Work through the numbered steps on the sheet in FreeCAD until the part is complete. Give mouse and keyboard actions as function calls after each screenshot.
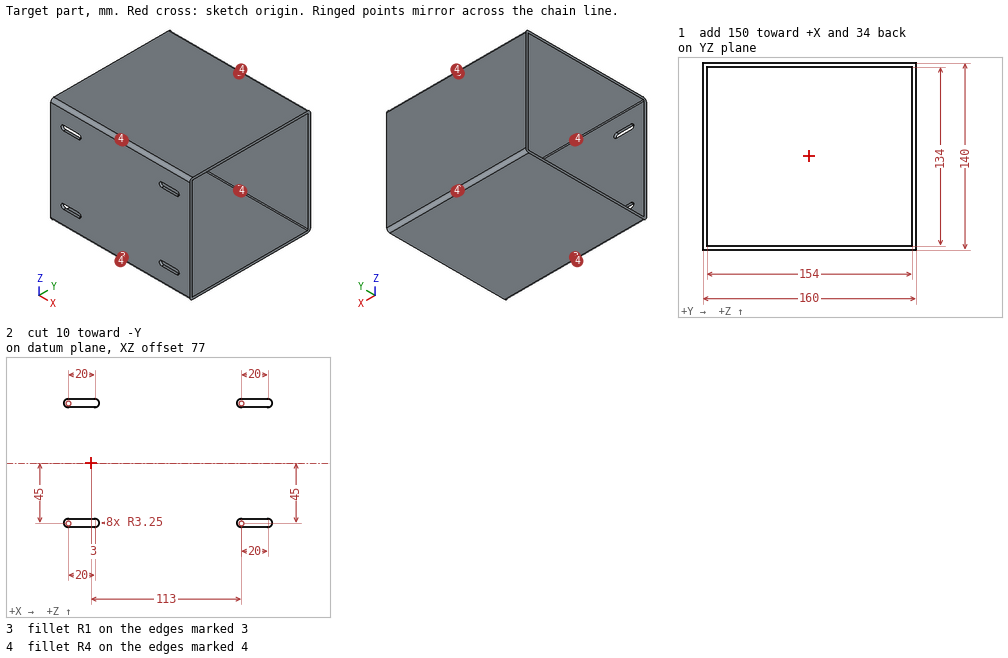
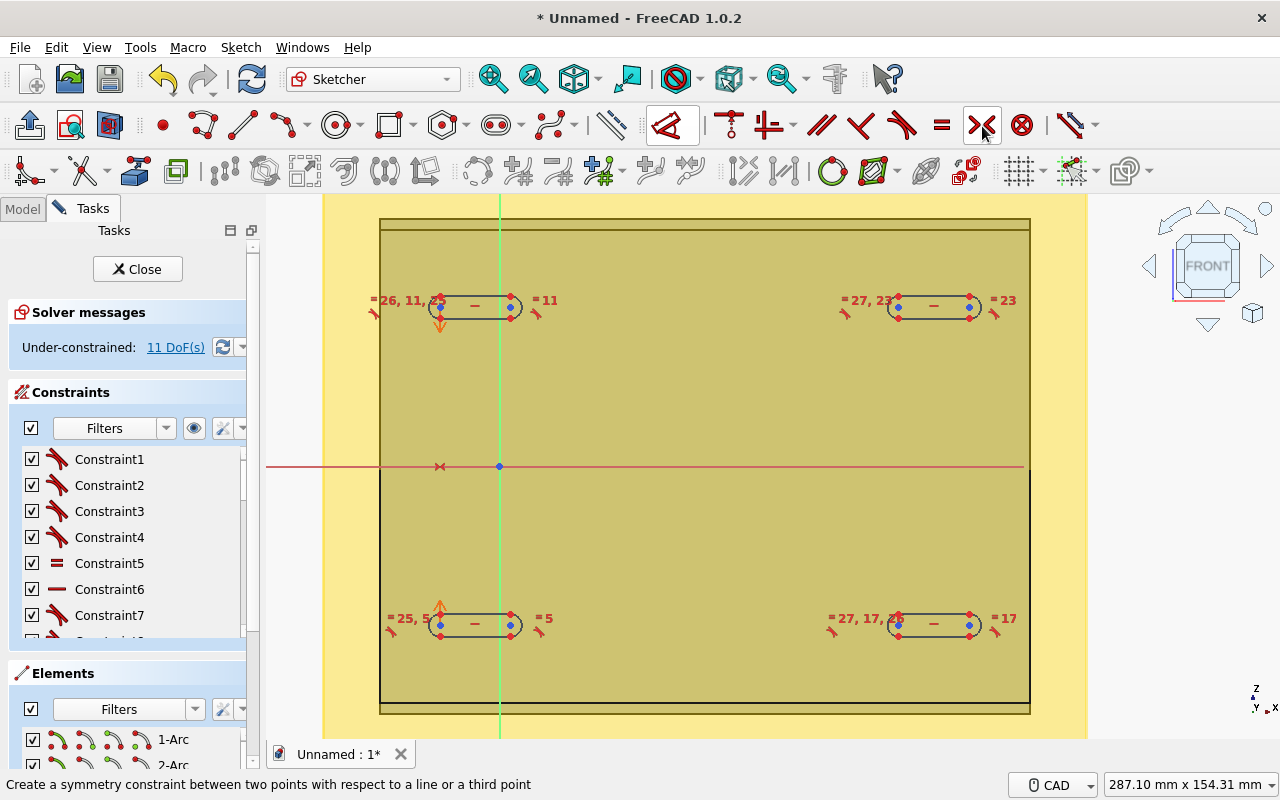
click(899, 625)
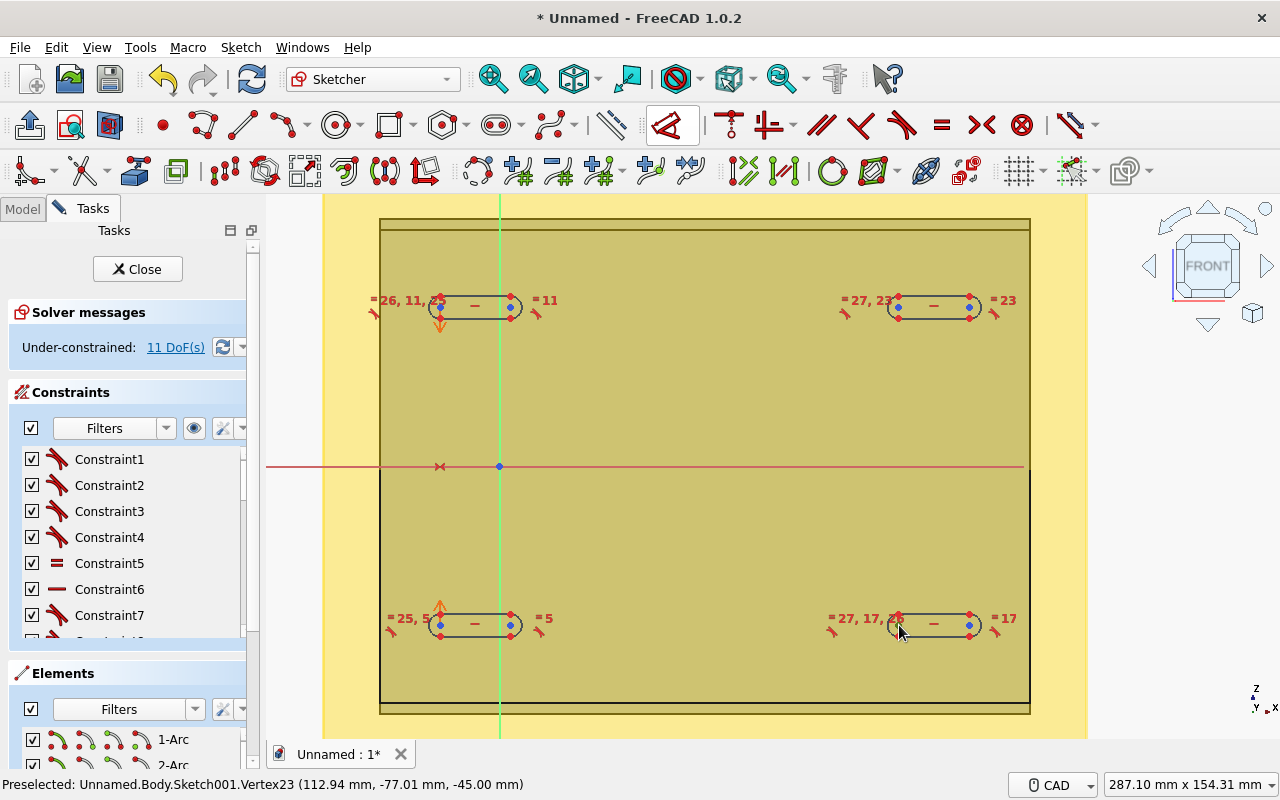
click(899, 308)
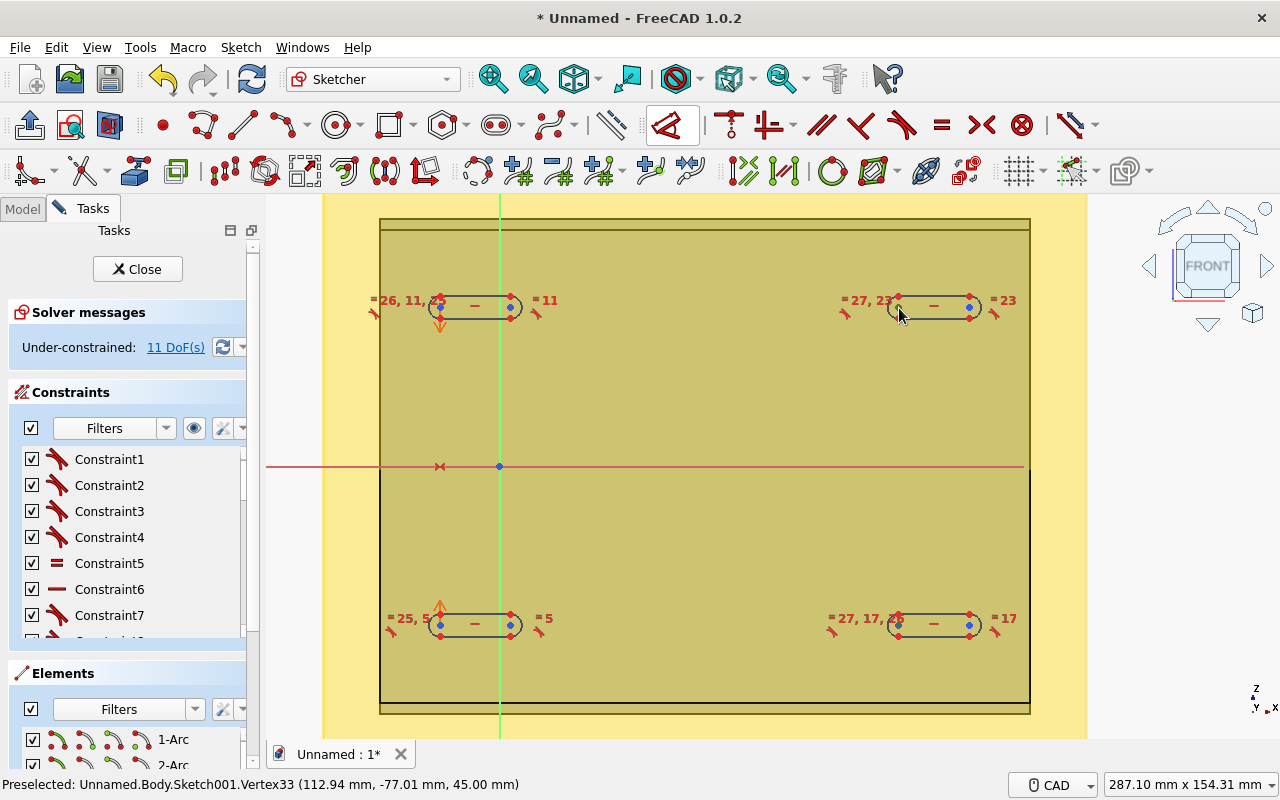
click(353, 466)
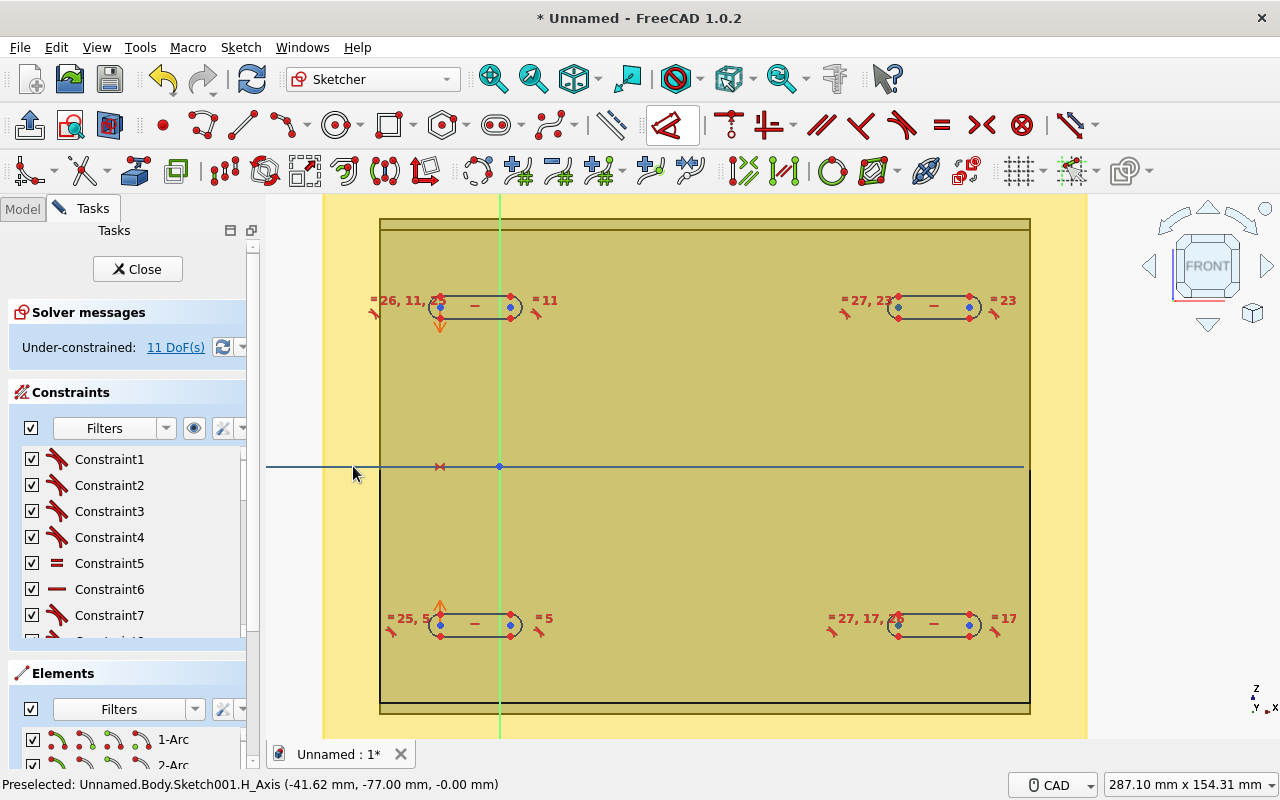
click(982, 126)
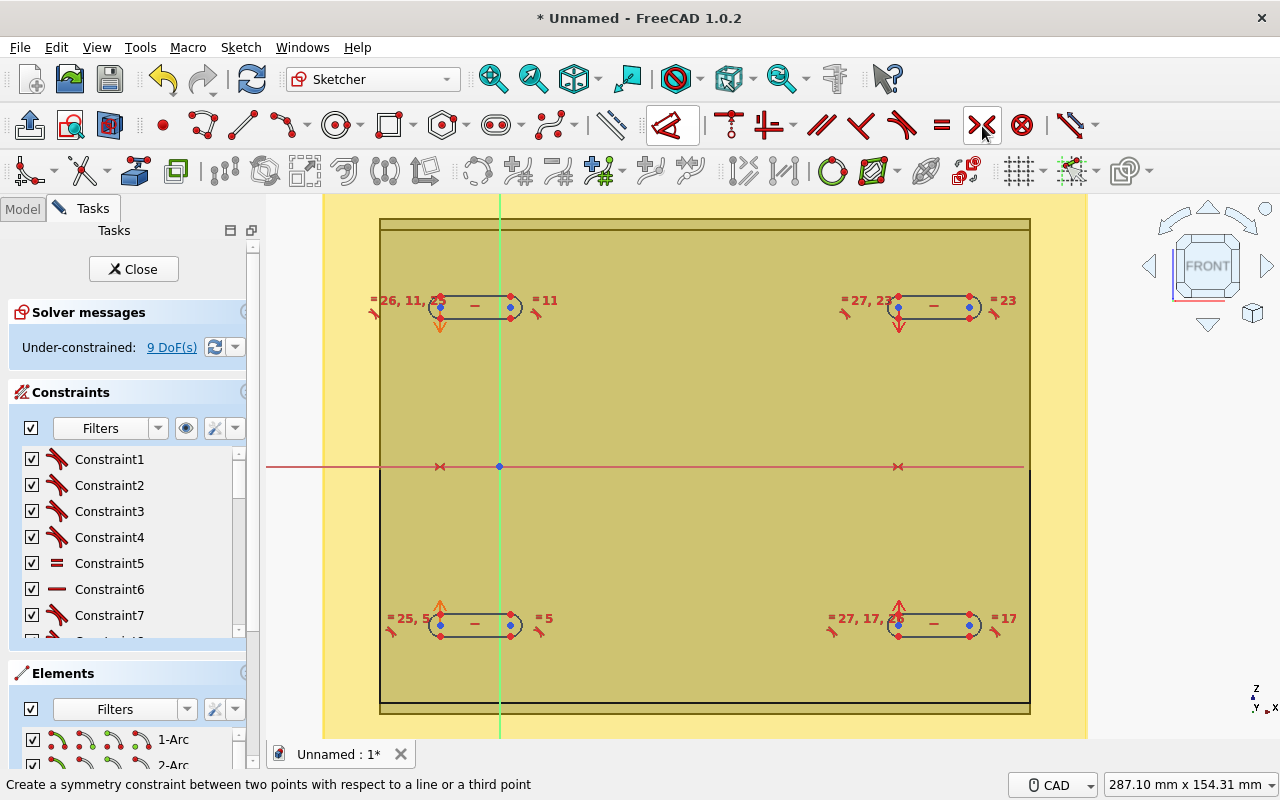
scroll(431, 619, up, 7)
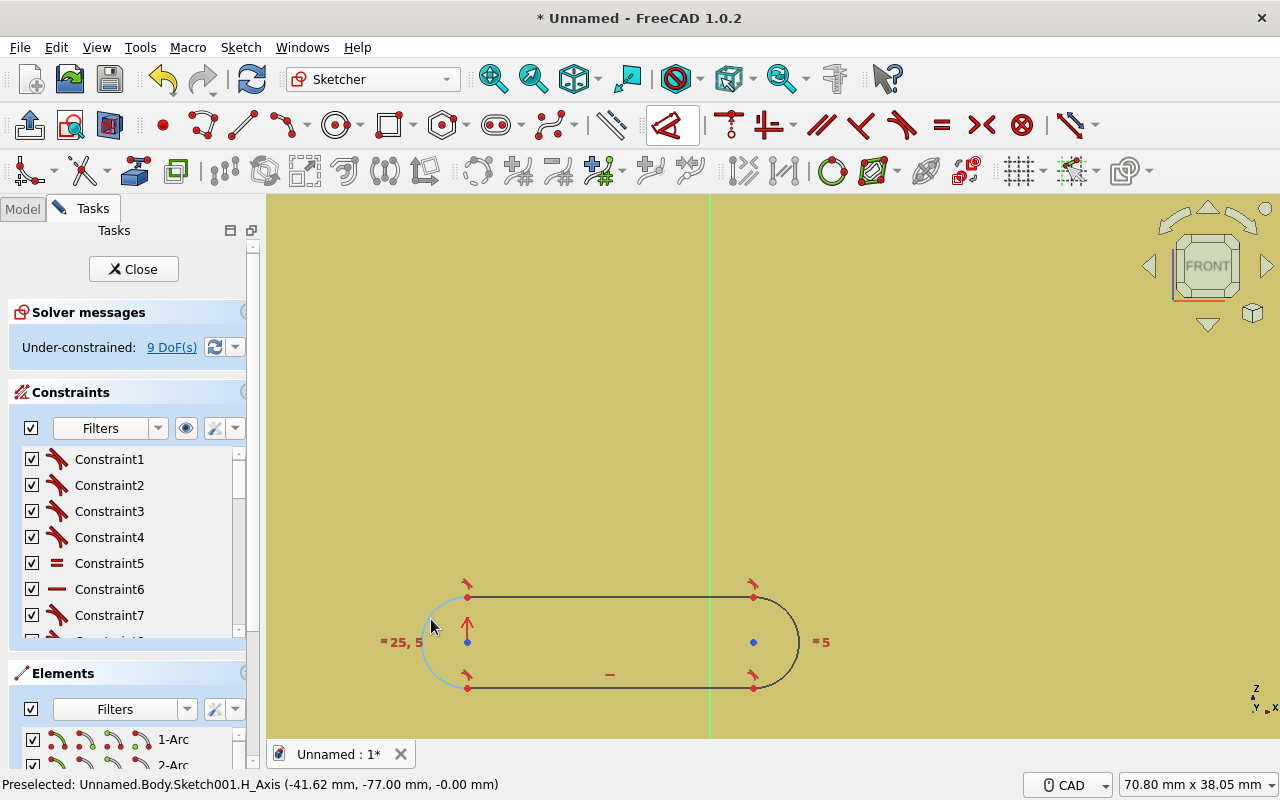
click(431, 616)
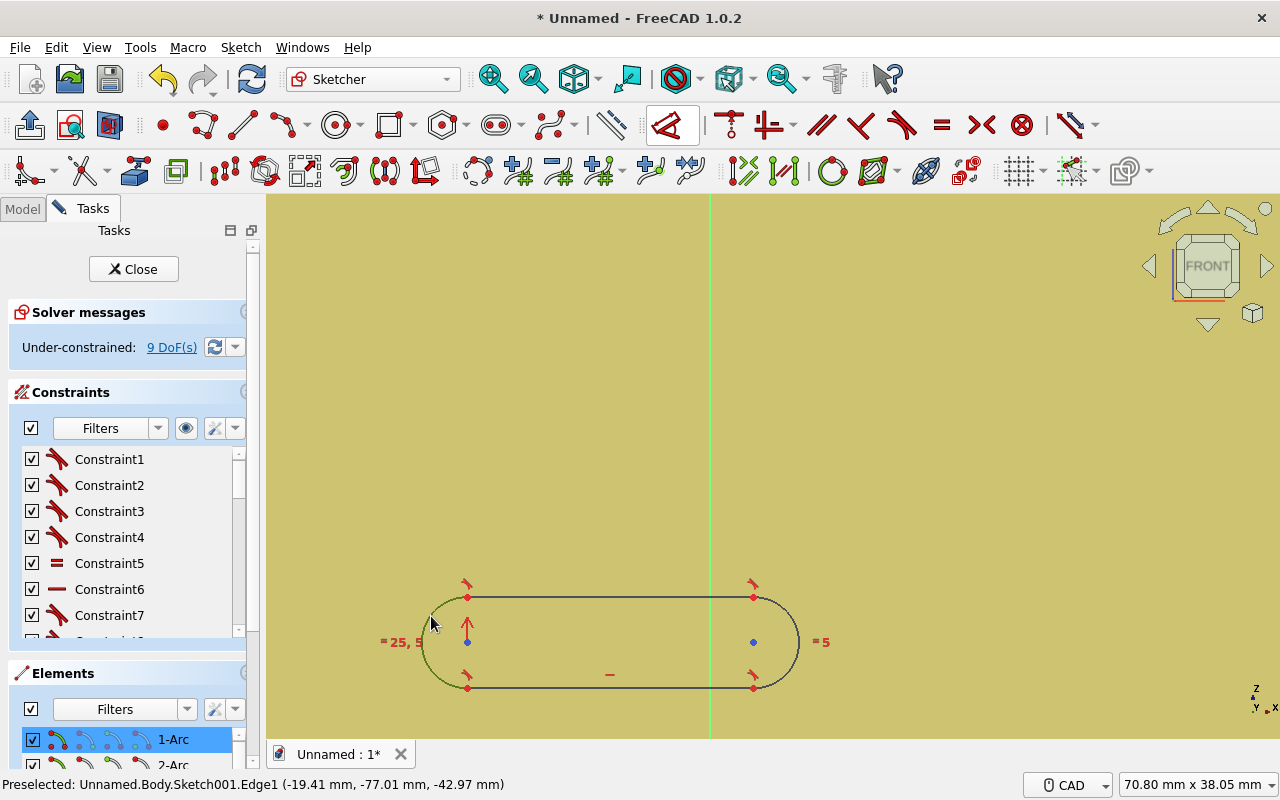
key(k)
key(r)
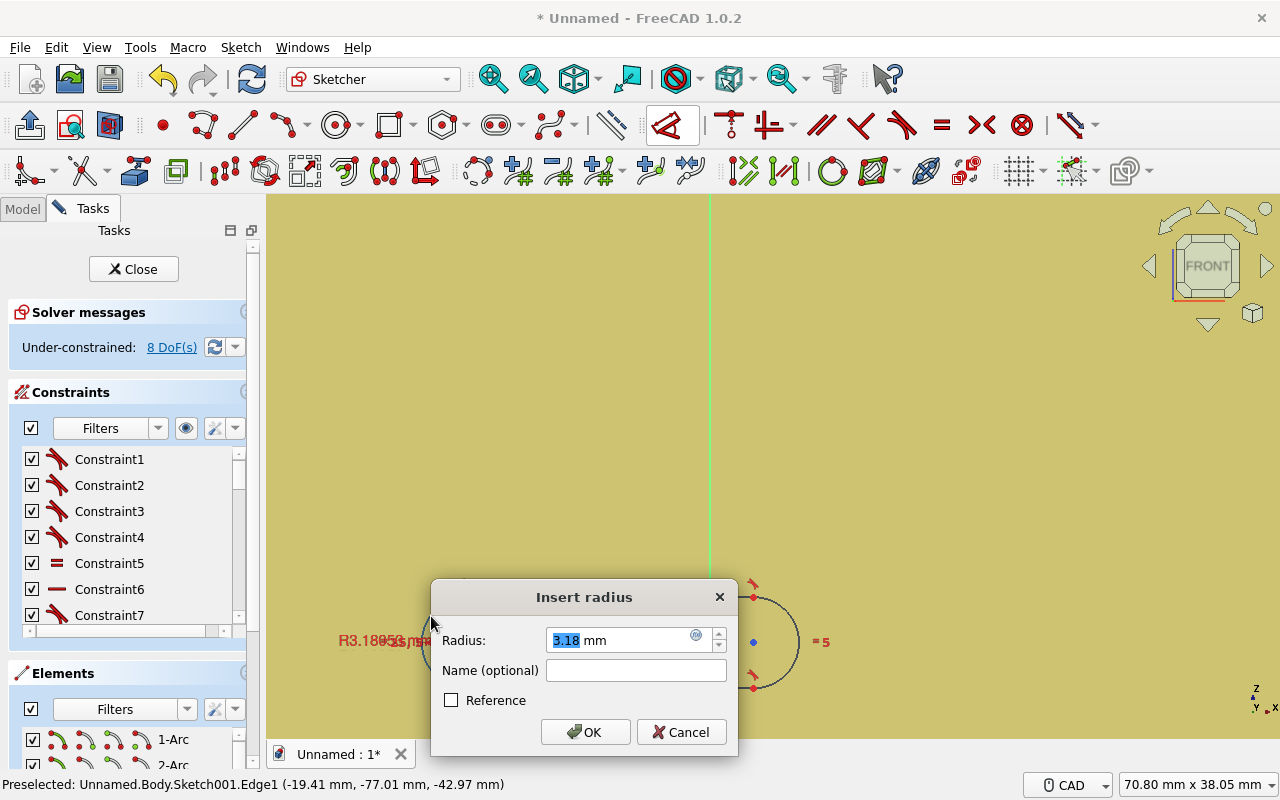
text(3.25)
key(Return)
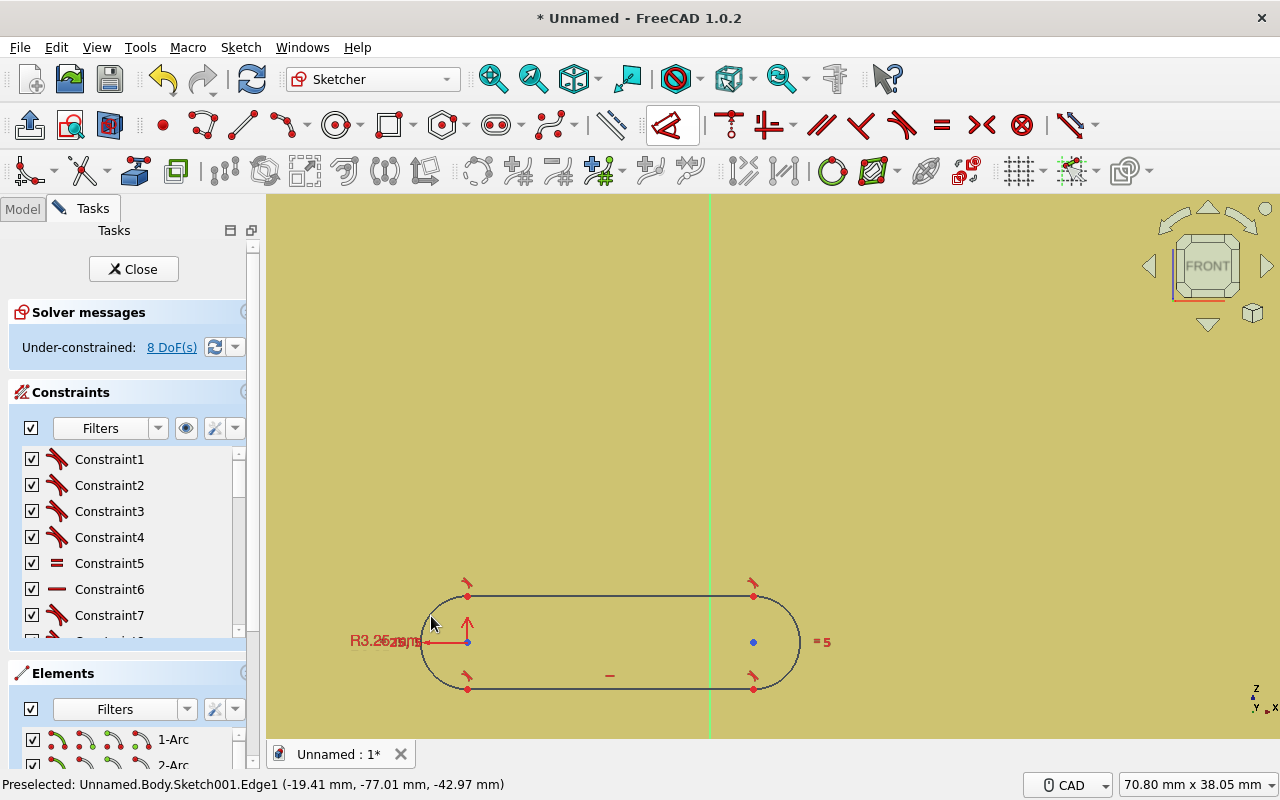
scroll(431, 620, down, 7)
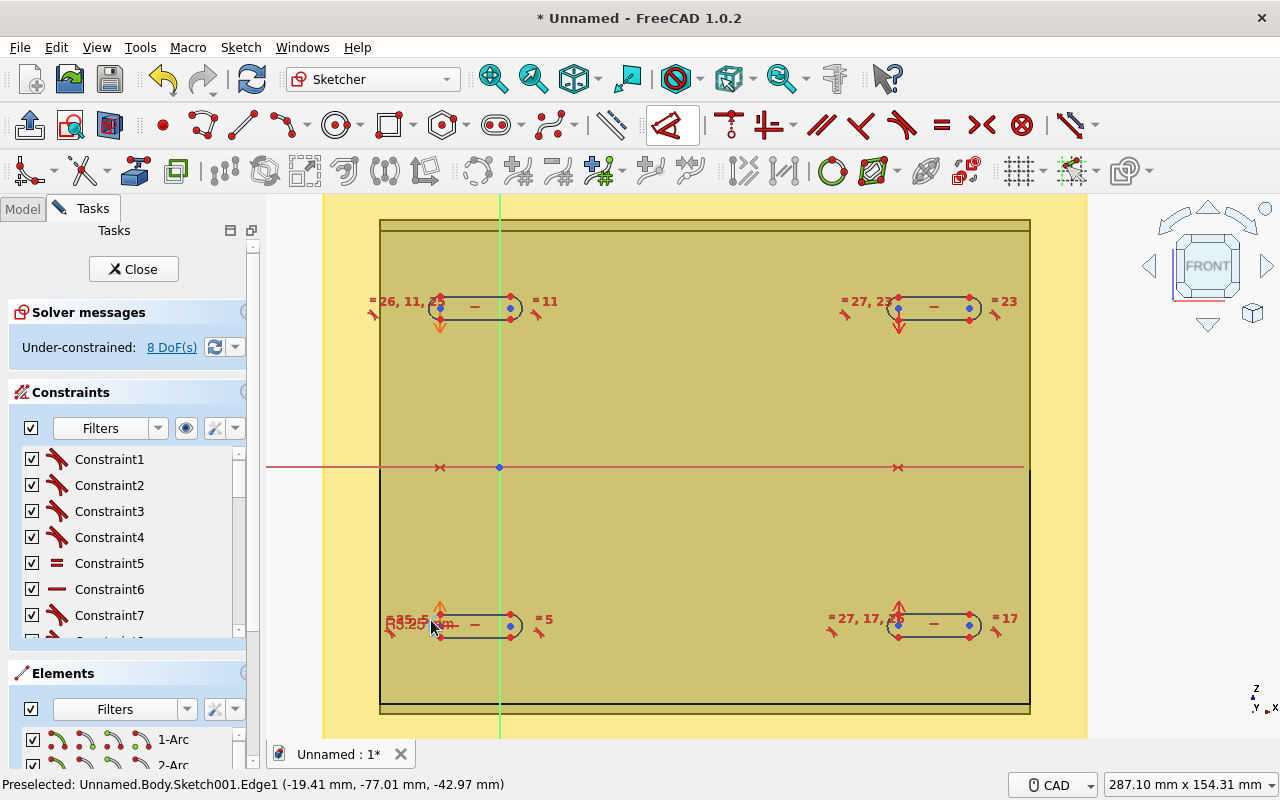
click(461, 615)